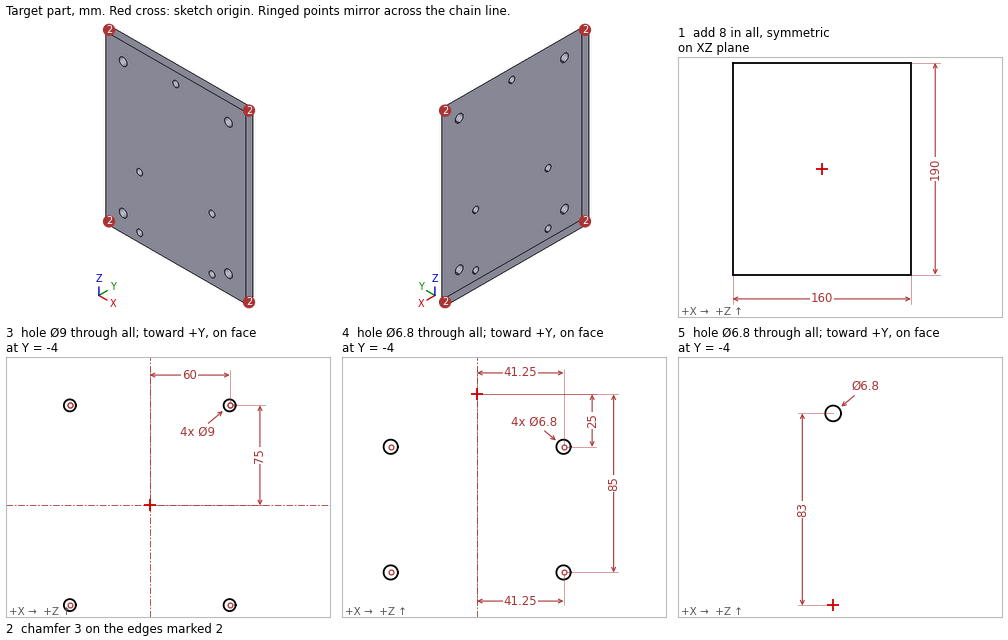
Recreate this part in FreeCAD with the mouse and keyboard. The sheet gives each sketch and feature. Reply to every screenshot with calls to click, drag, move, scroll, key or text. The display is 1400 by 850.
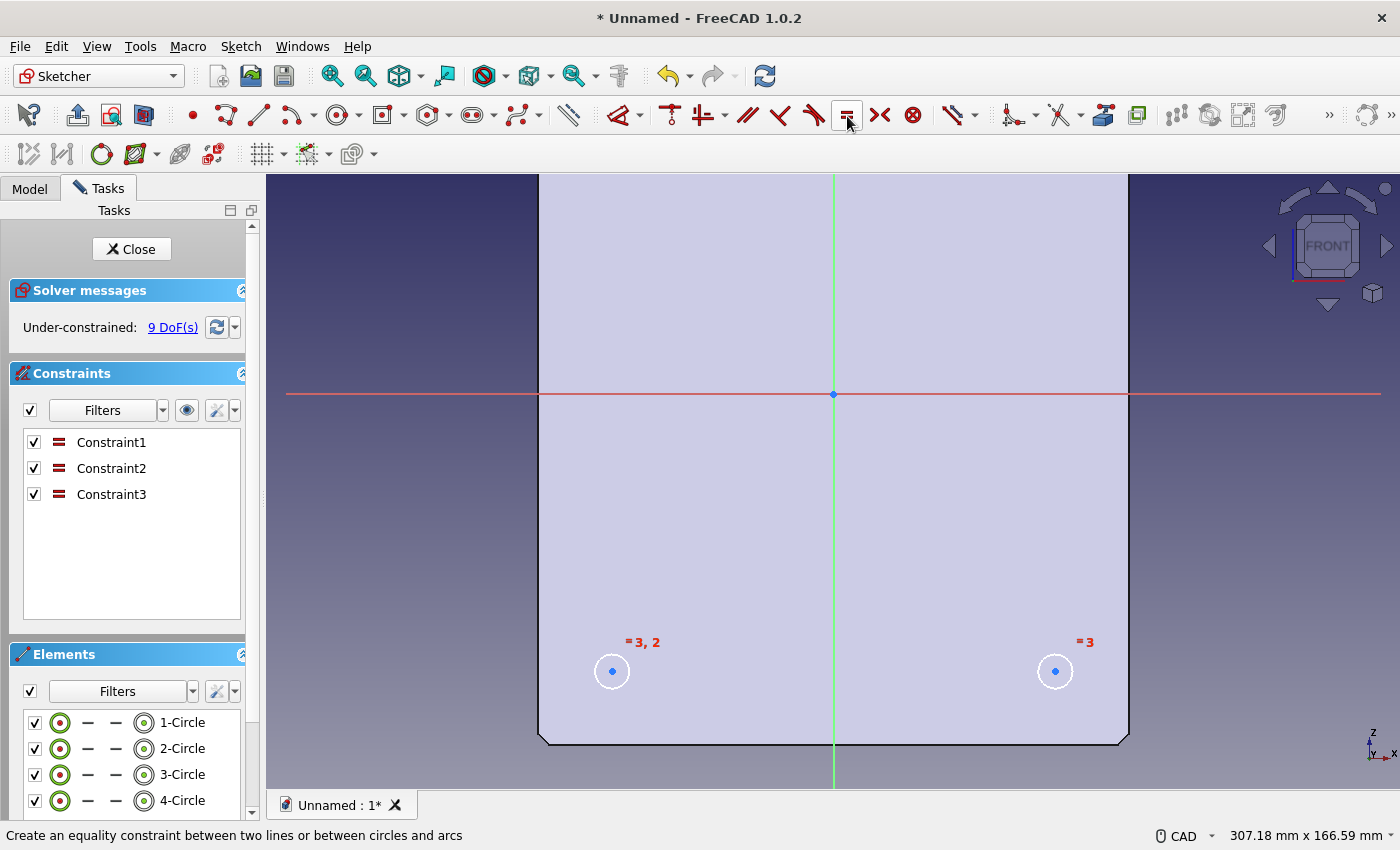
scroll(624, 659, down, 2)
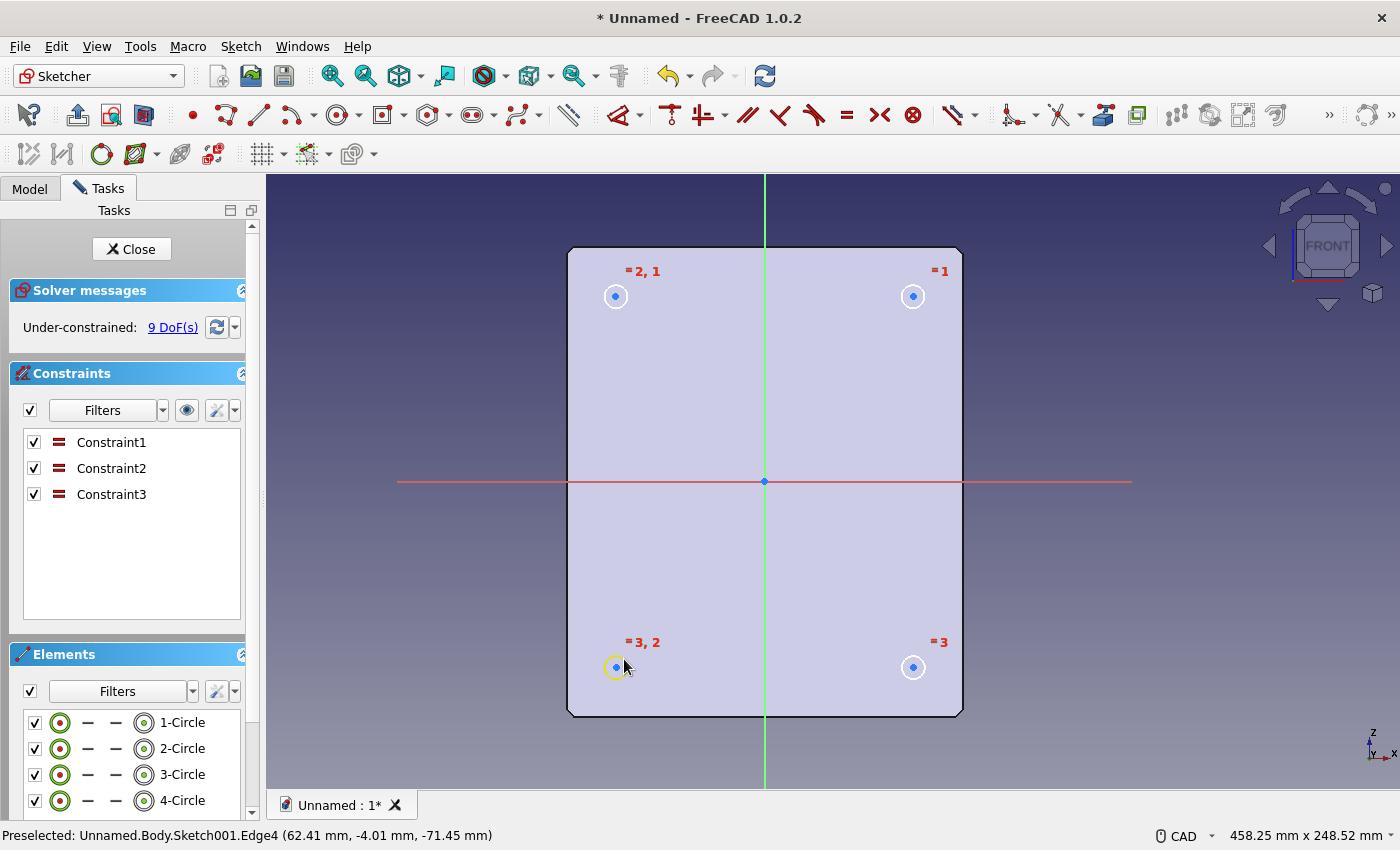
click(913, 297)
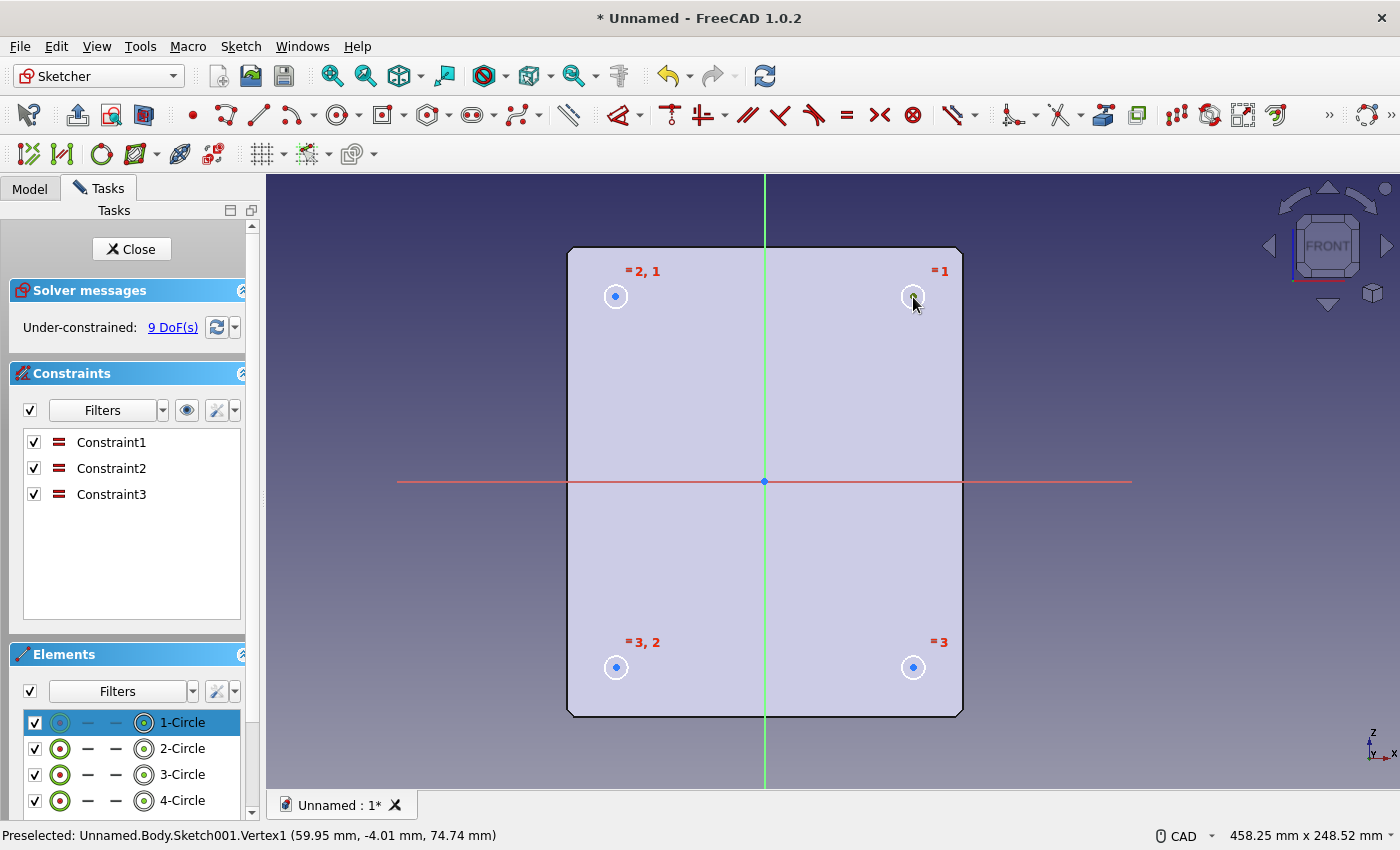
click(616, 297)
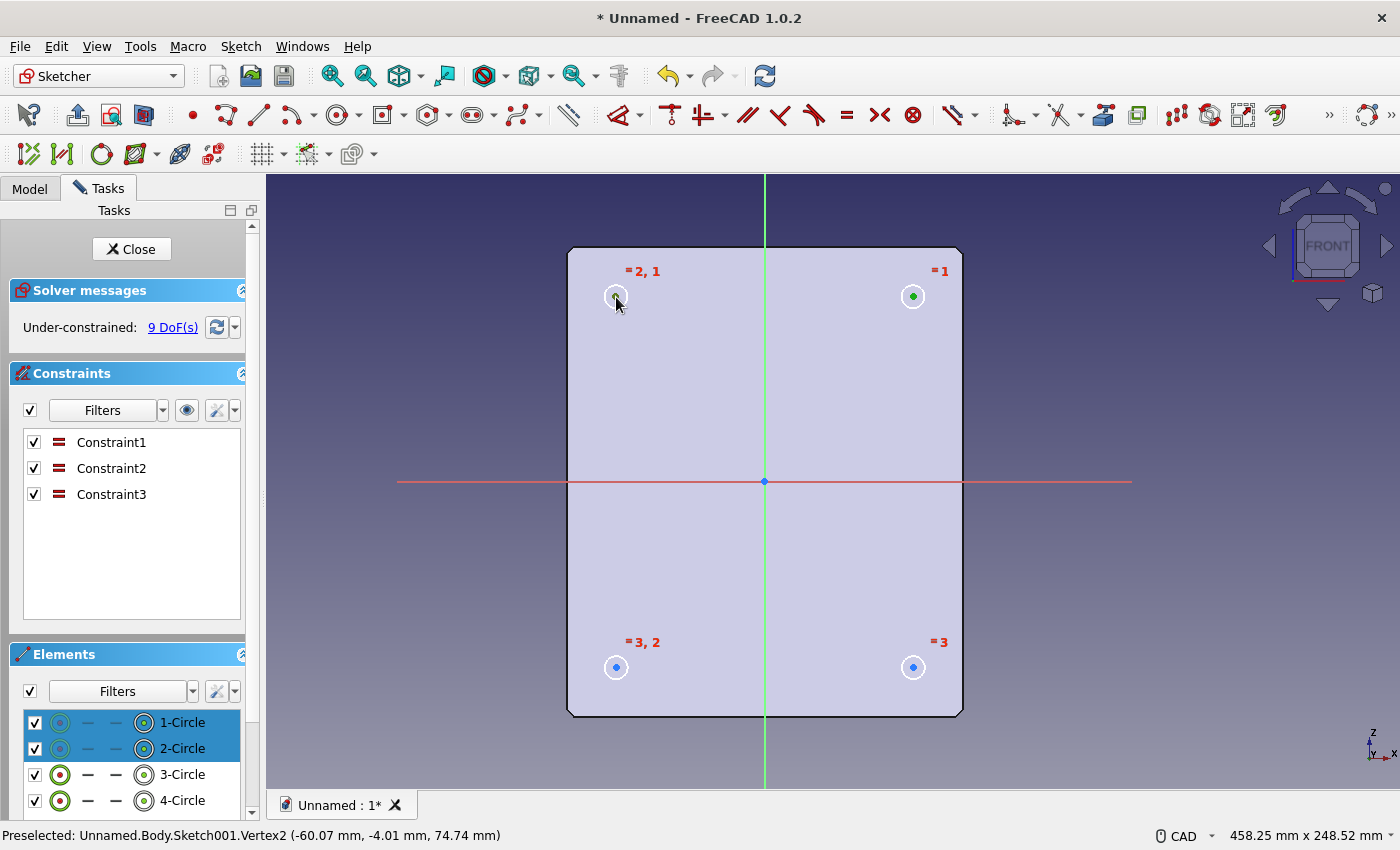
click(765, 721)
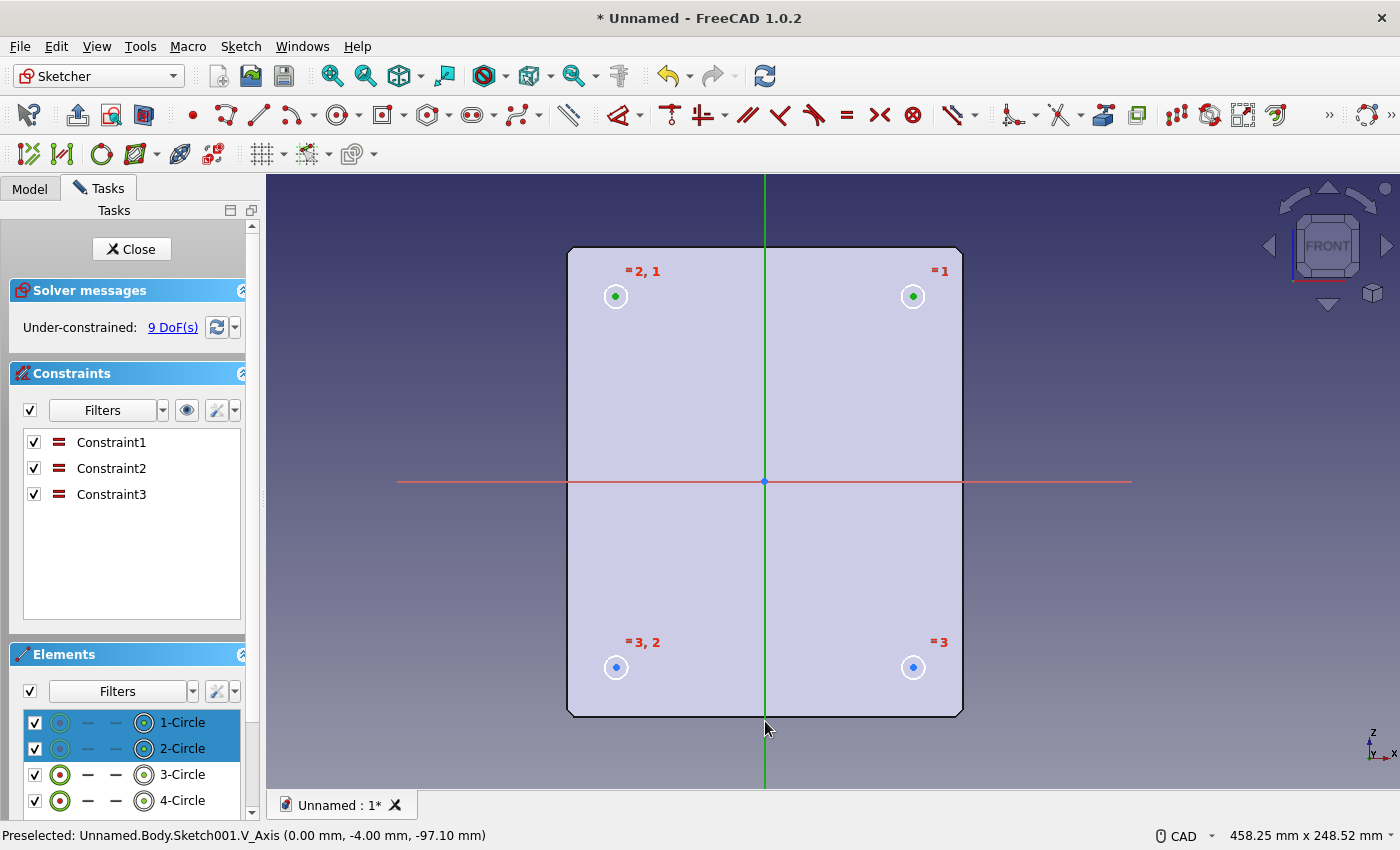
click(880, 116)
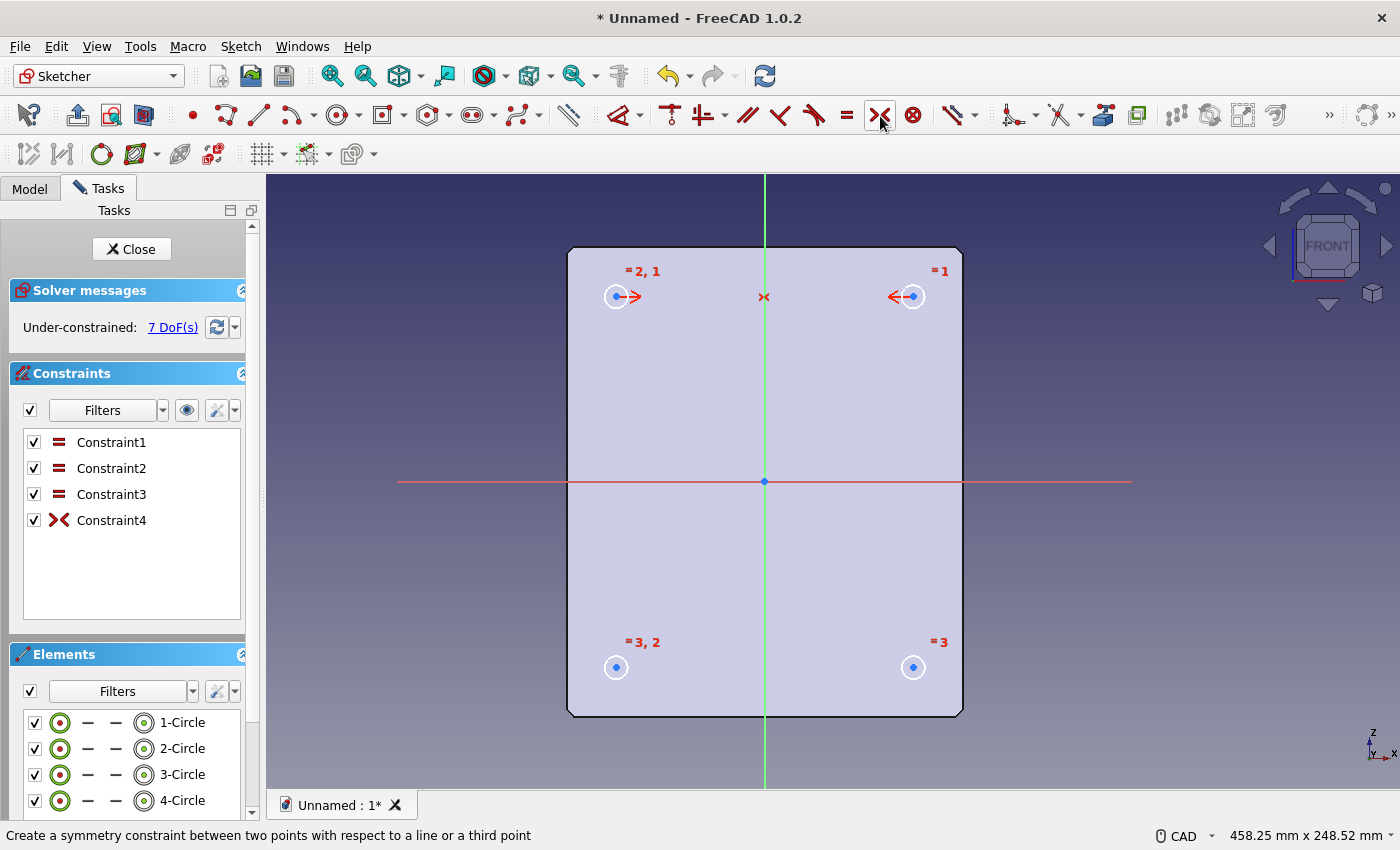
click(616, 297)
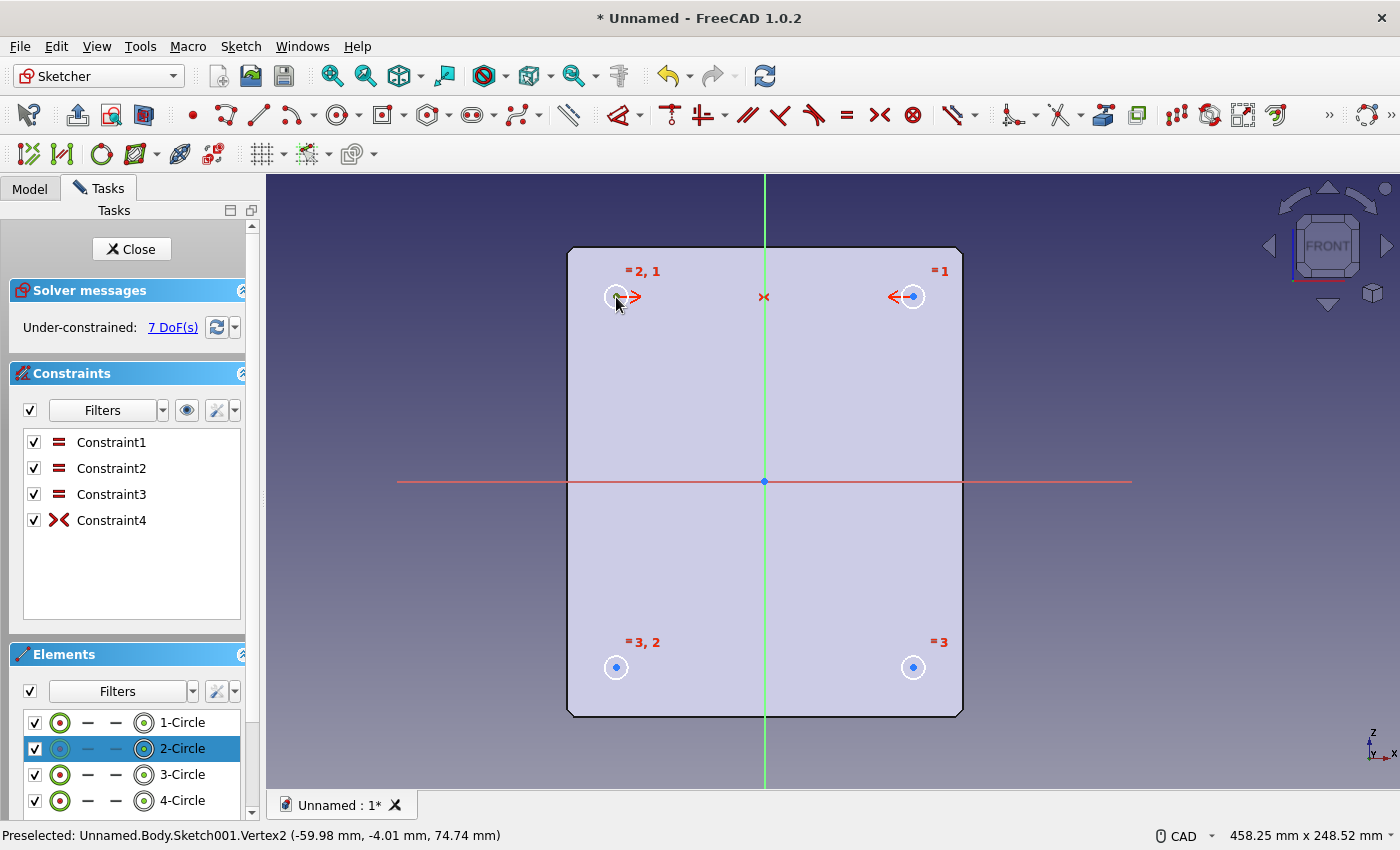
click(616, 668)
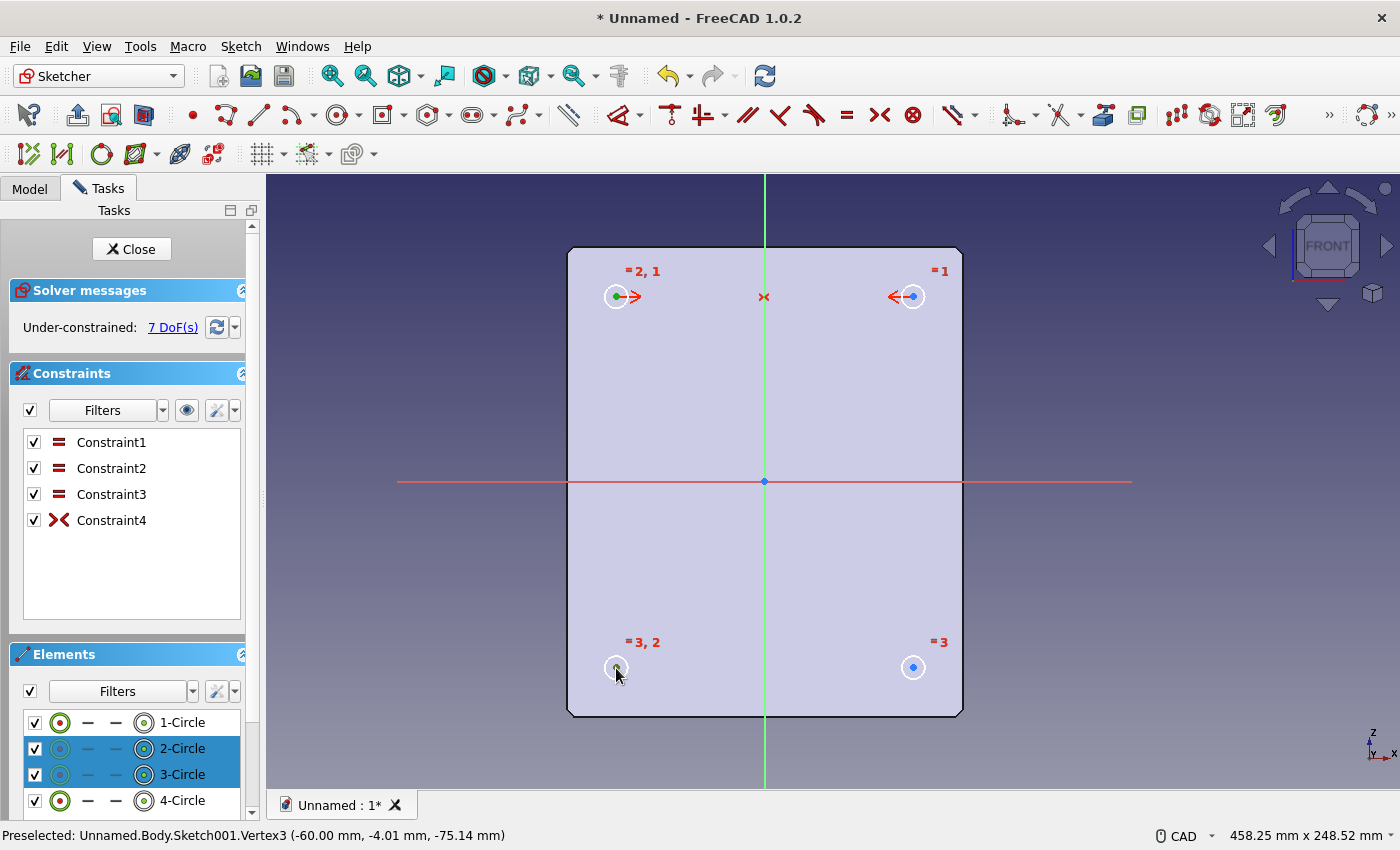
click(428, 482)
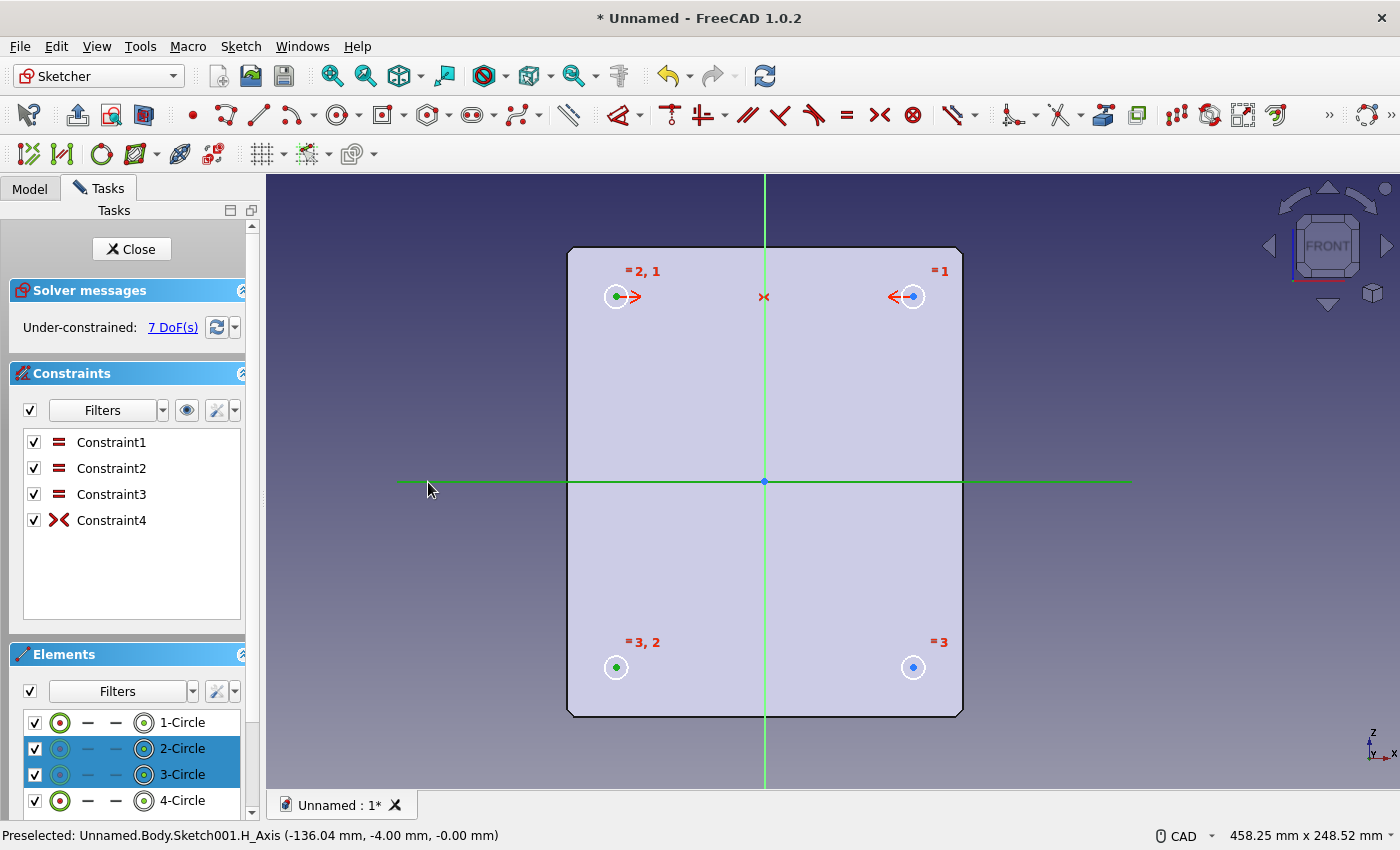
click(880, 116)